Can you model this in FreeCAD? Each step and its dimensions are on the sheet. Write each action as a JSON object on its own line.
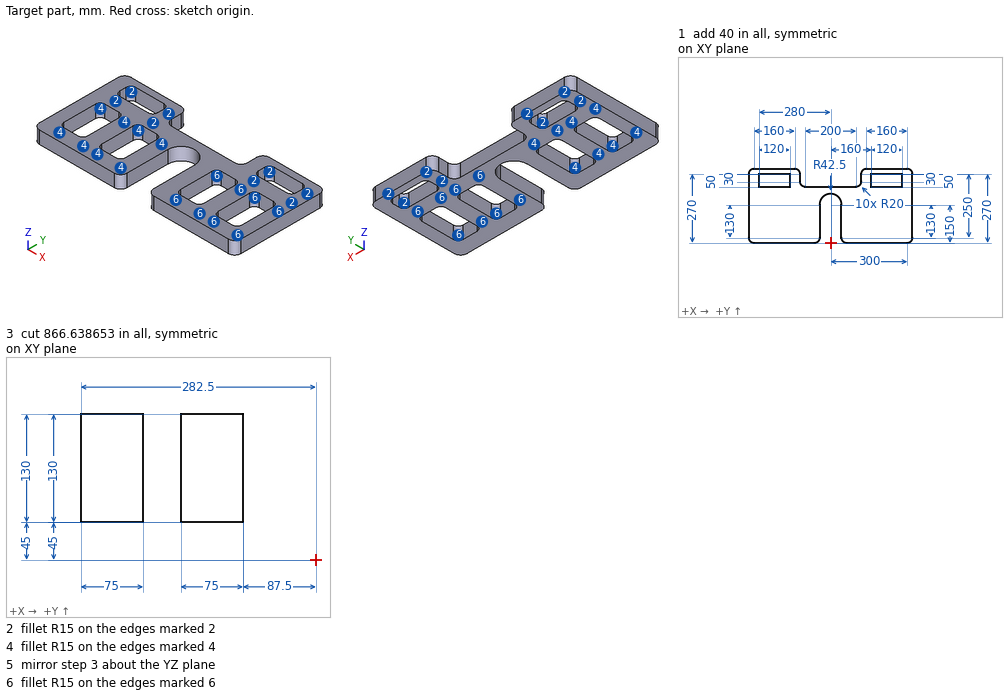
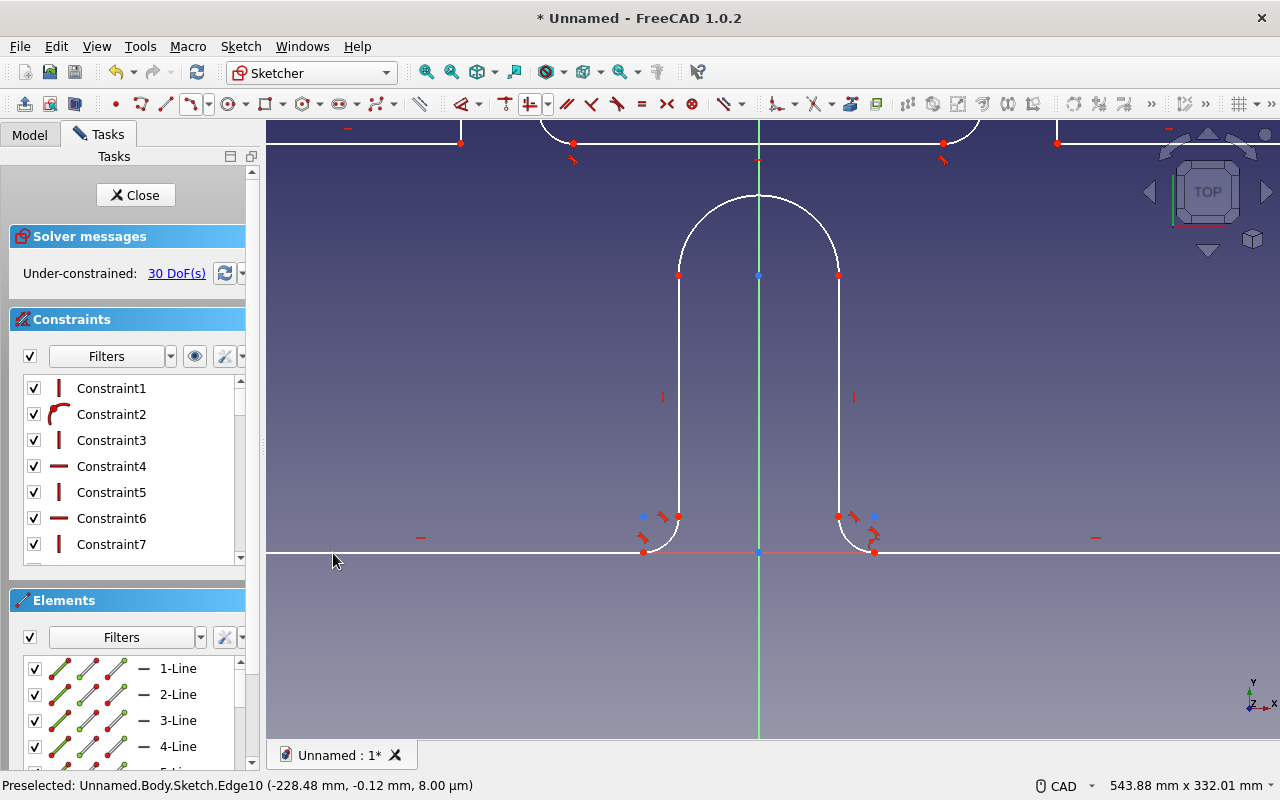
{"action": "left_click", "coordinate": [843, 533]}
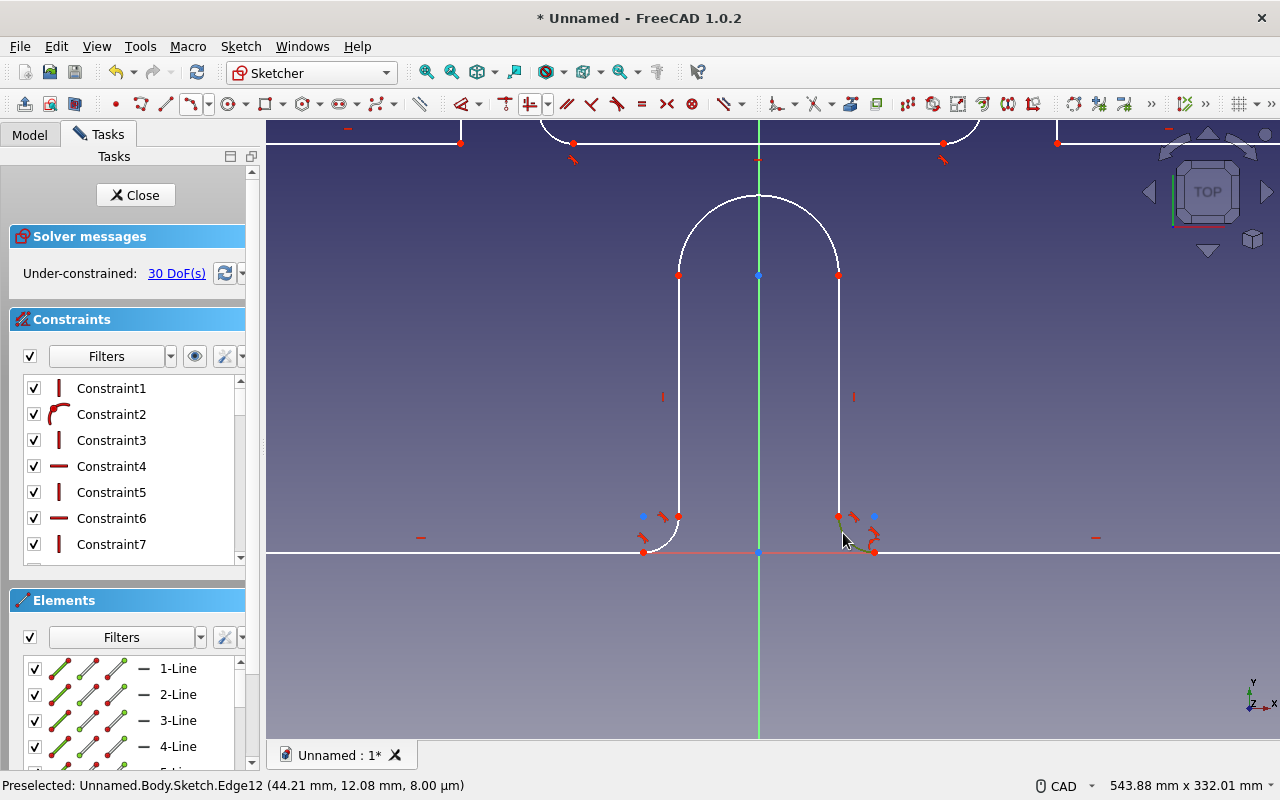
{"action": "scroll", "coordinate": [660, 550], "scroll_direction": "down", "scroll_amount": 4}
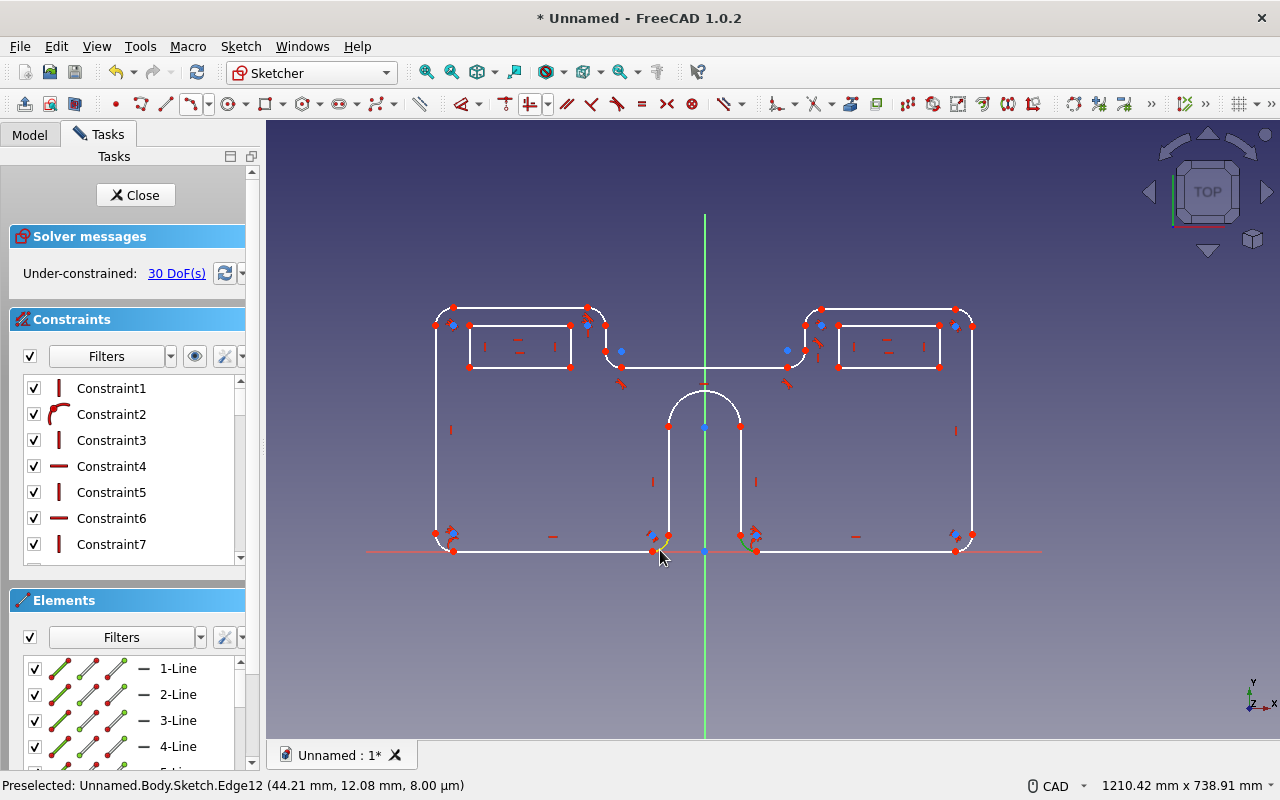
{"action": "scroll", "coordinate": [971, 542], "scroll_direction": "up", "scroll_amount": 3}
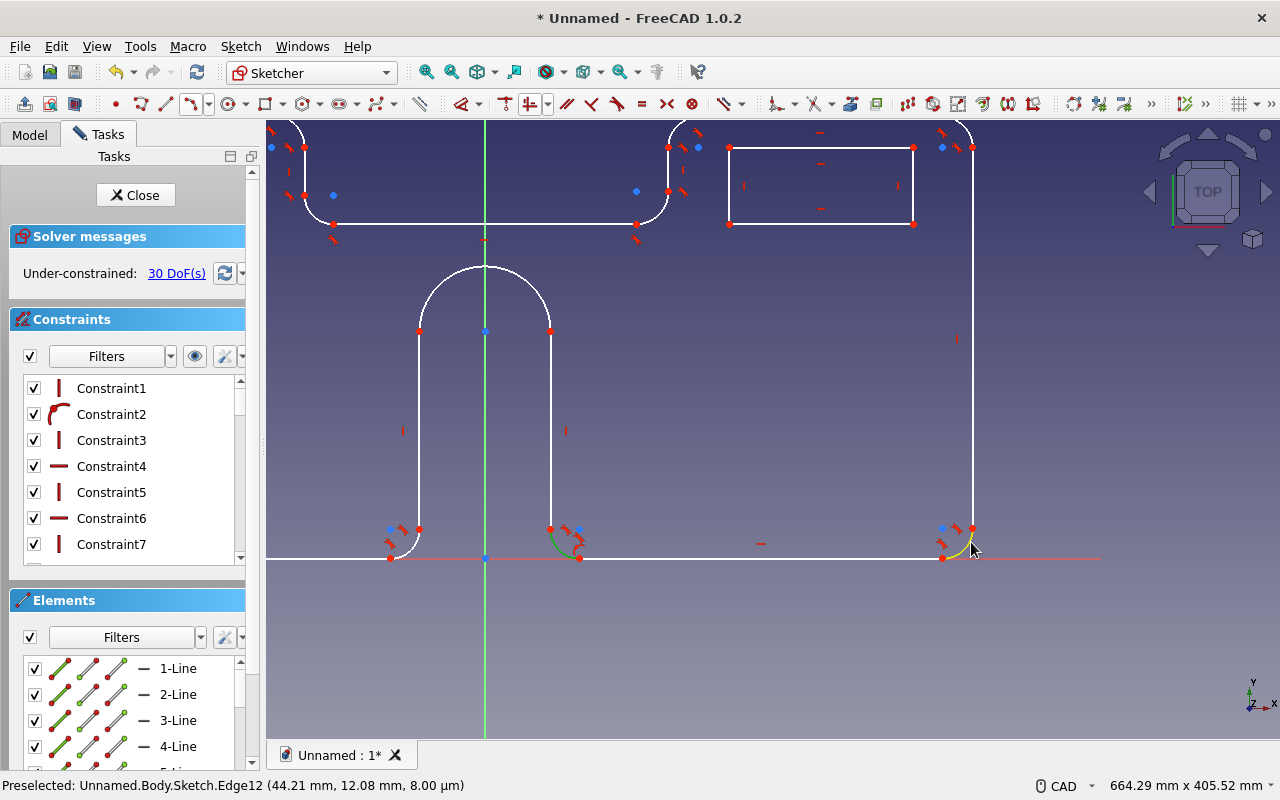
{"action": "left_click", "coordinate": [970, 542]}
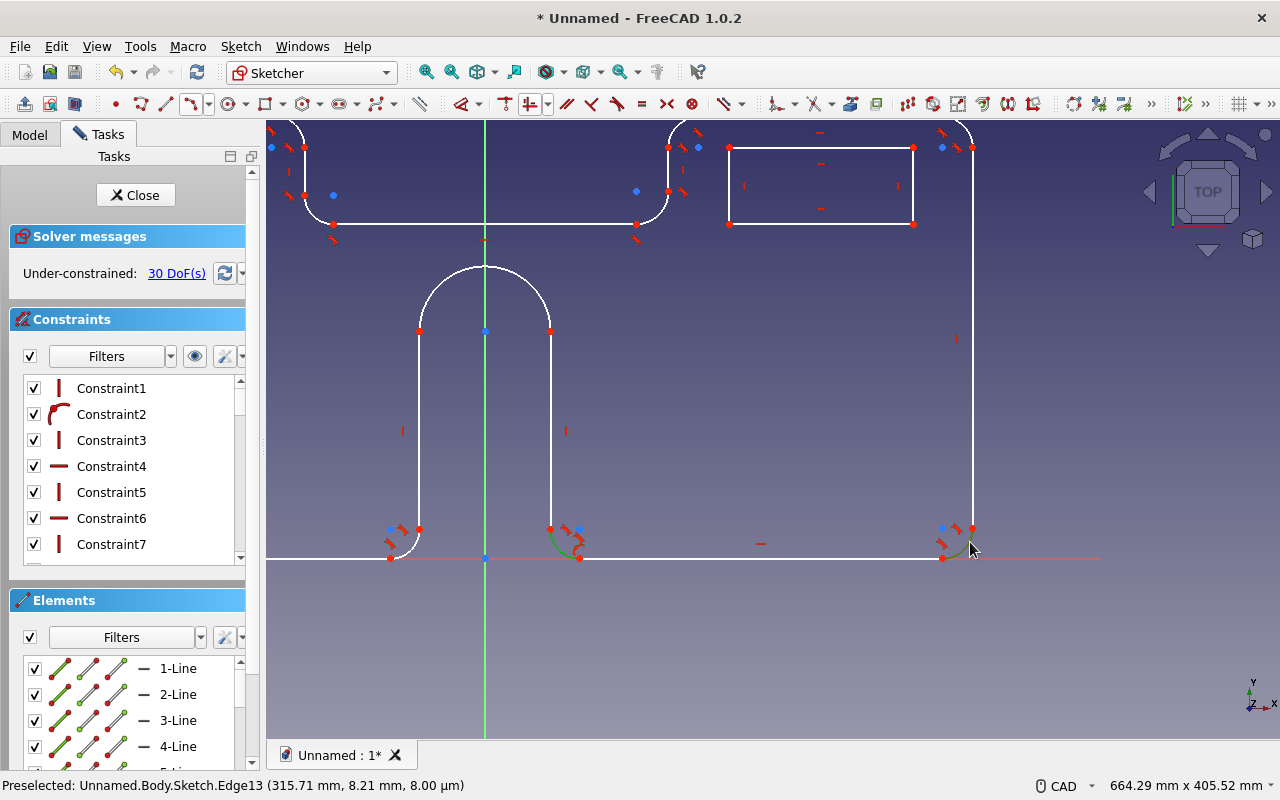
{"action": "scroll", "coordinate": [971, 541], "scroll_direction": "down", "scroll_amount": 3}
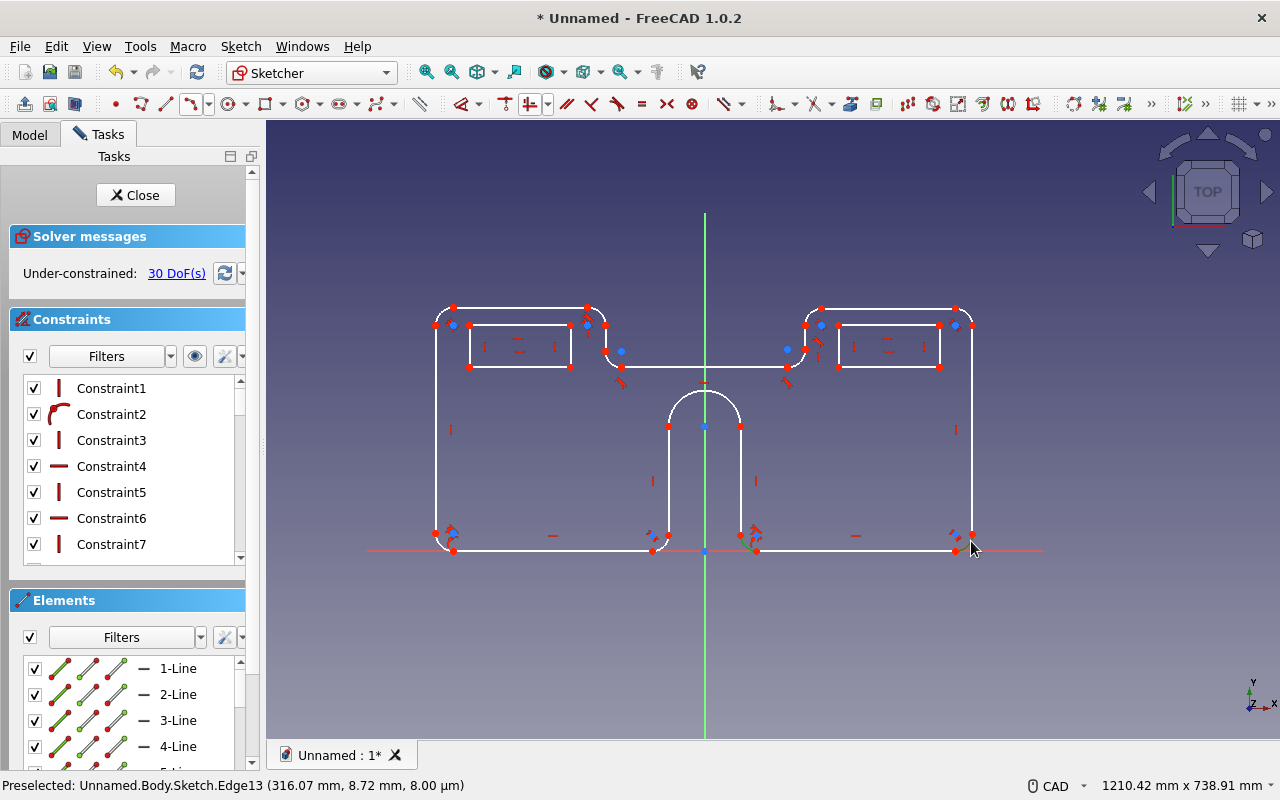
{"action": "scroll", "coordinate": [971, 318], "scroll_direction": "up", "scroll_amount": 3}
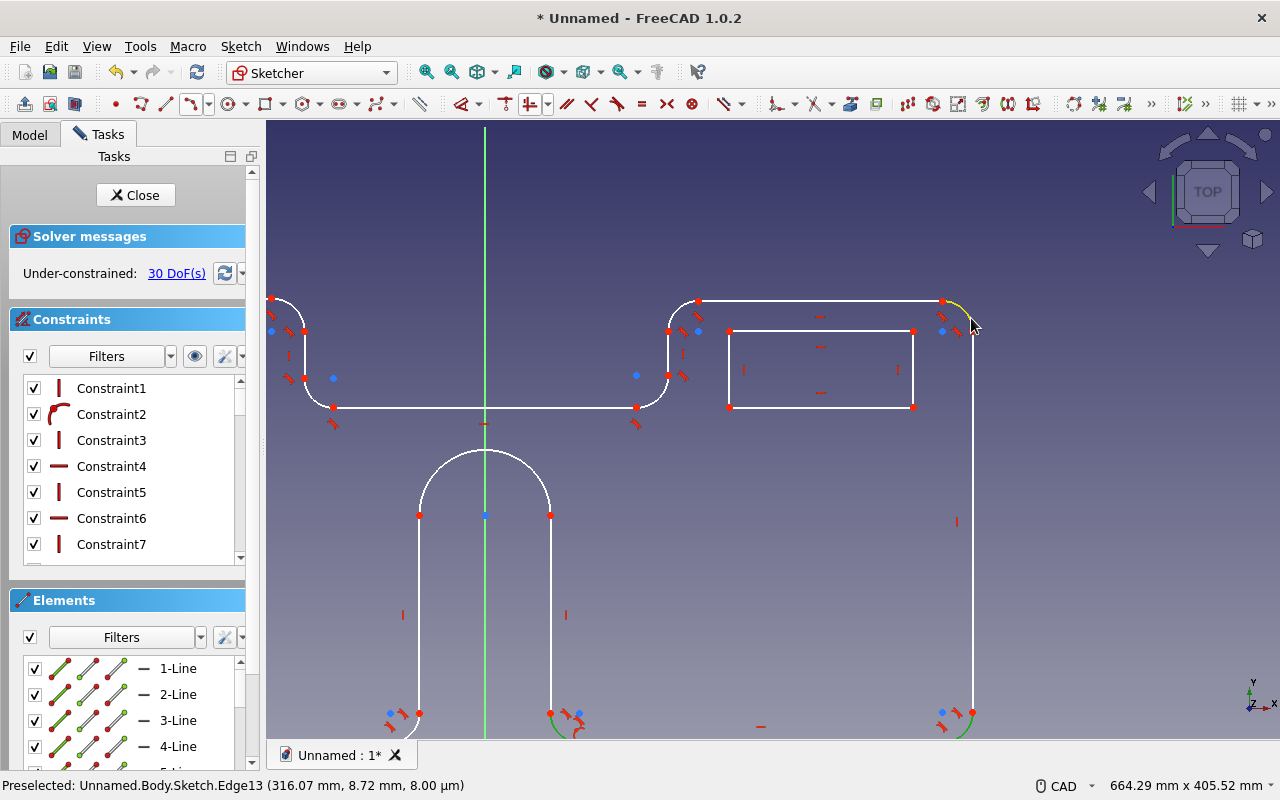
{"action": "left_click", "coordinate": [970, 318]}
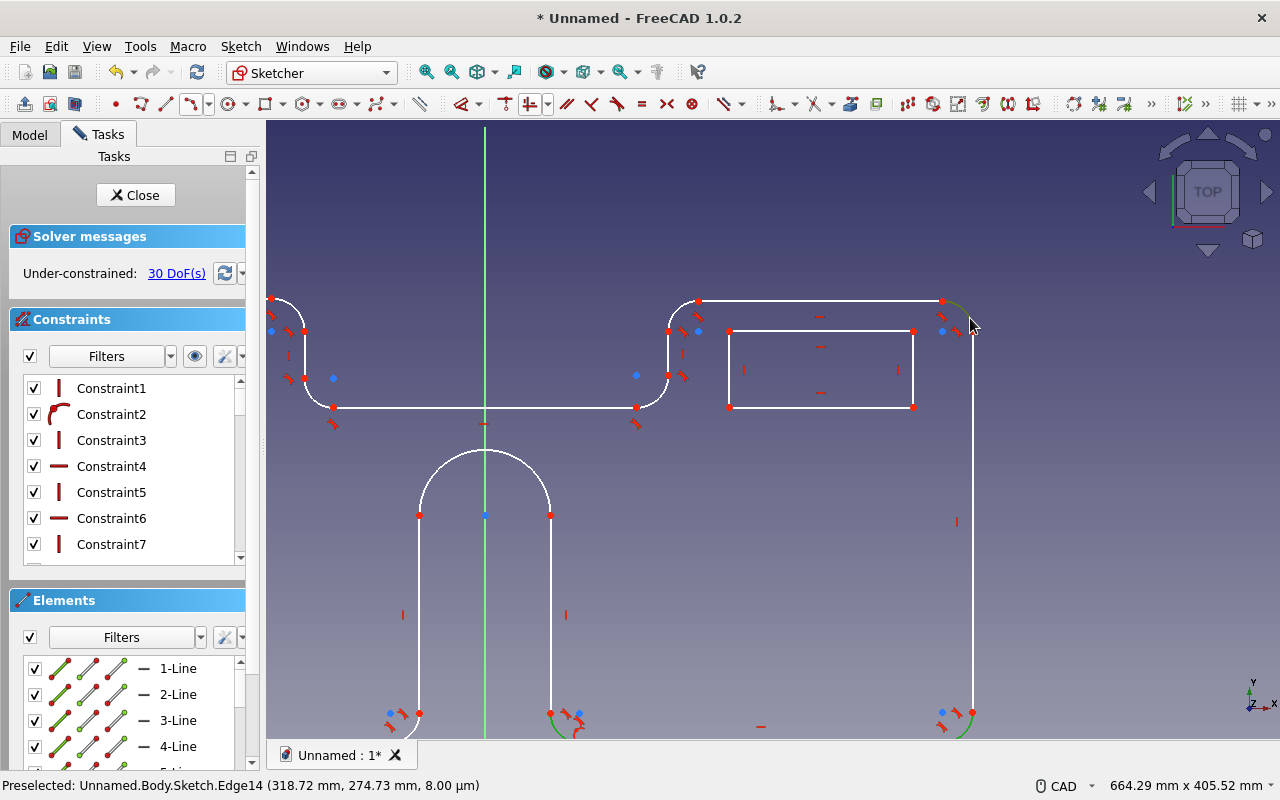
{"action": "left_click", "coordinate": [685, 304]}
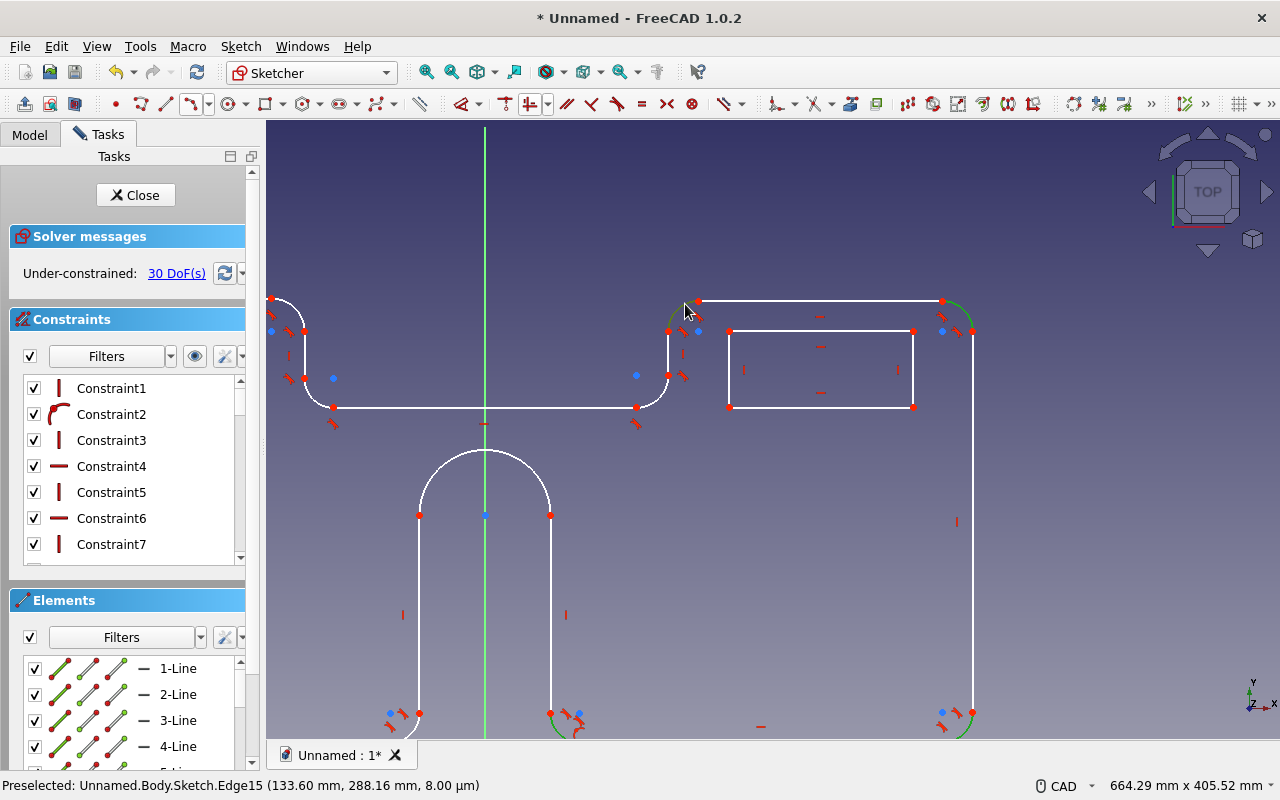
{"action": "left_click", "coordinate": [651, 404]}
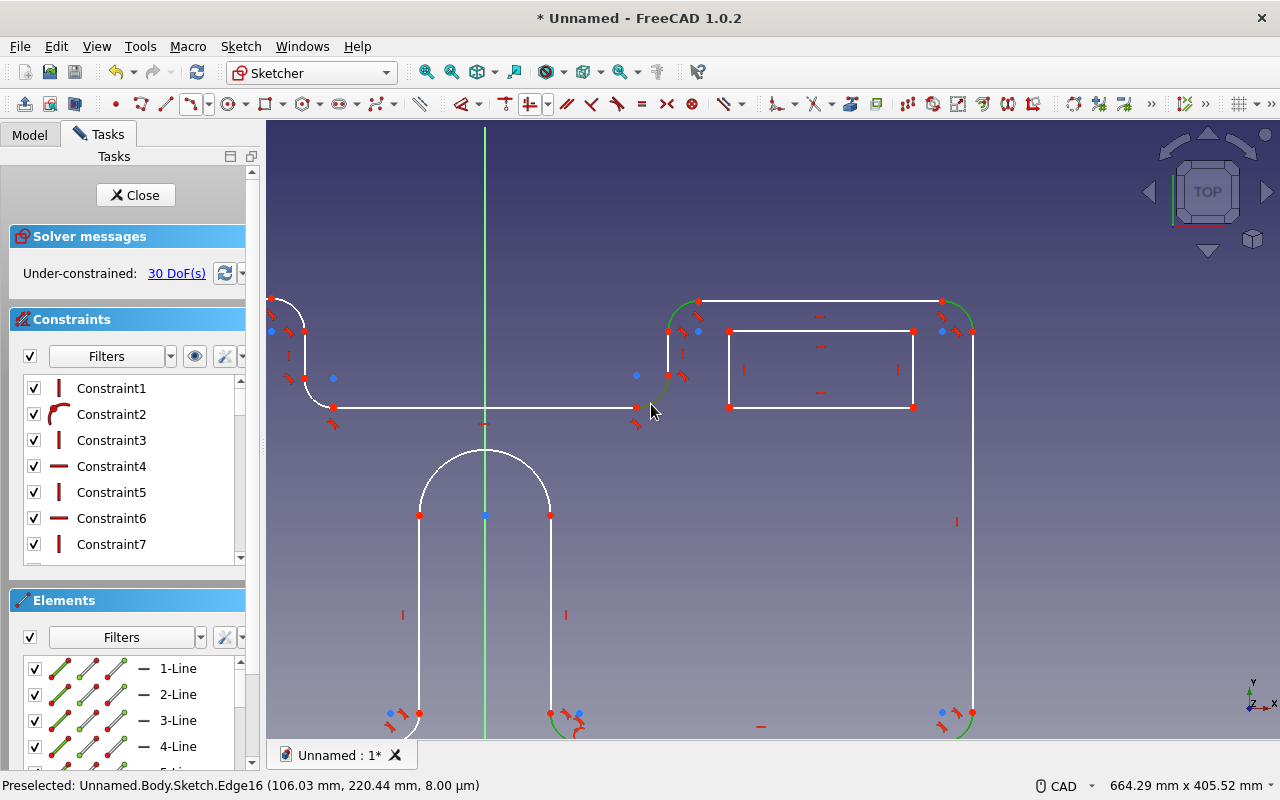
{"action": "left_click", "coordinate": [308, 392]}